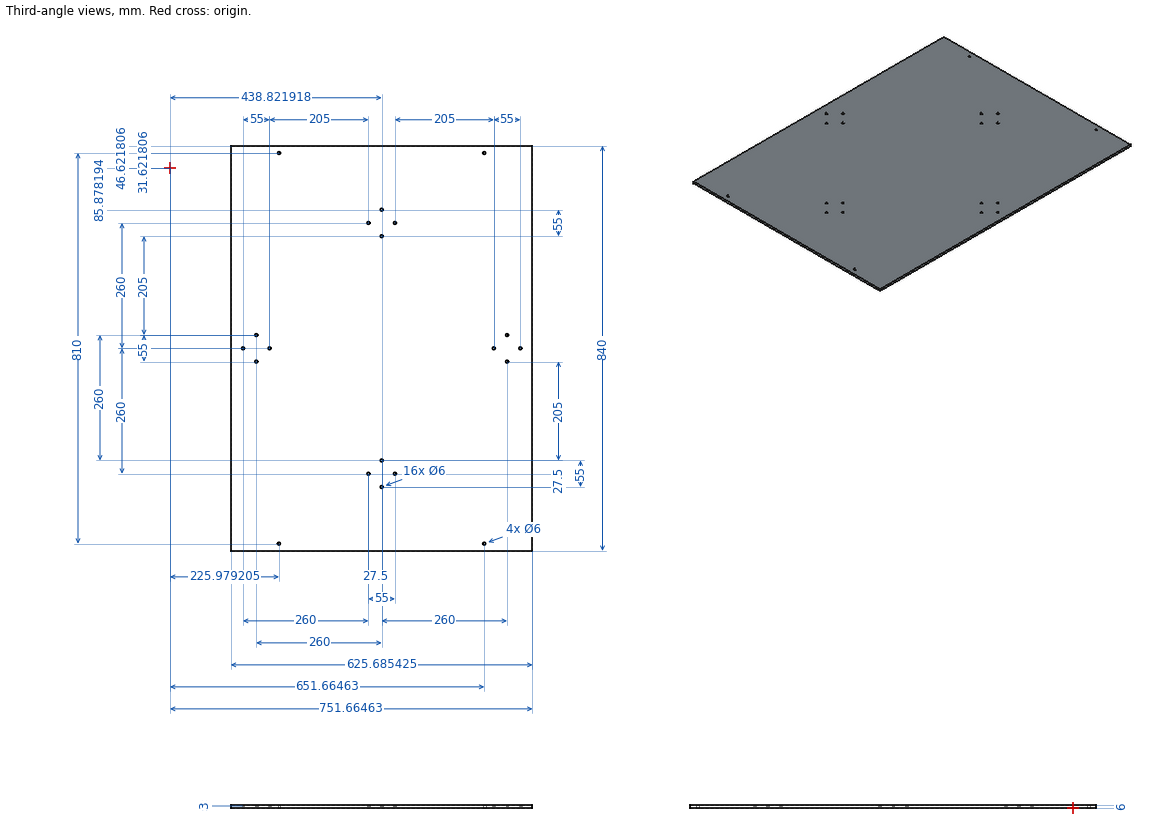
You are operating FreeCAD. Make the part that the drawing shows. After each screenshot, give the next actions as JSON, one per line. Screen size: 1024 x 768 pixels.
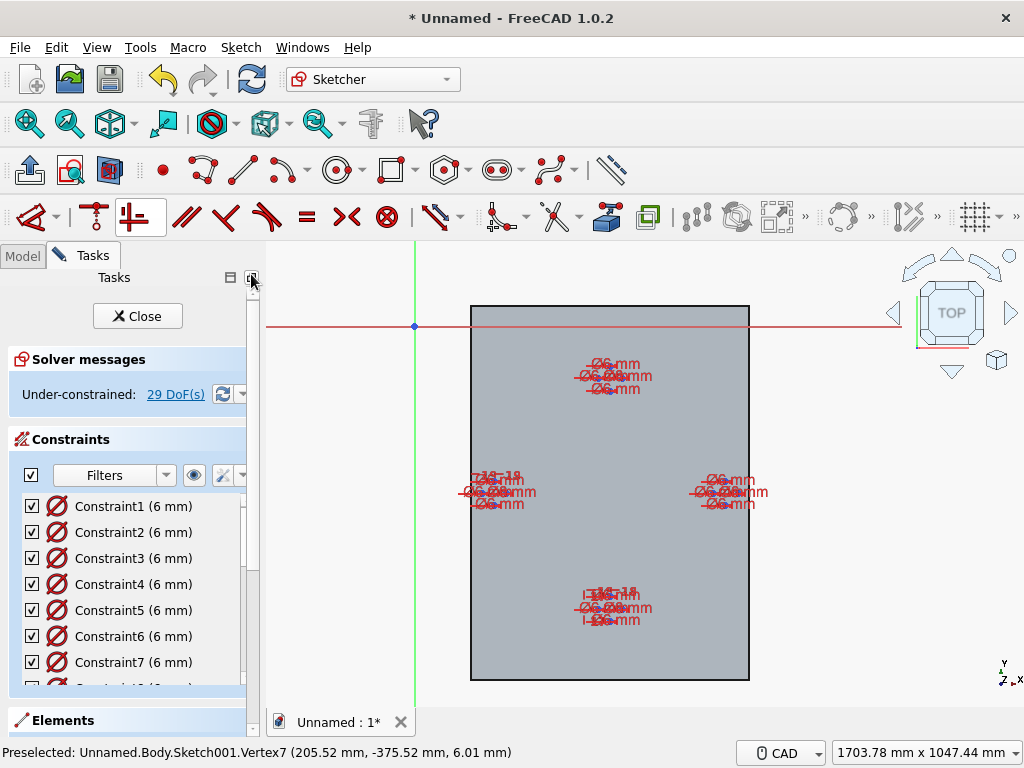
{"action": "left_click", "coordinate": [494, 482]}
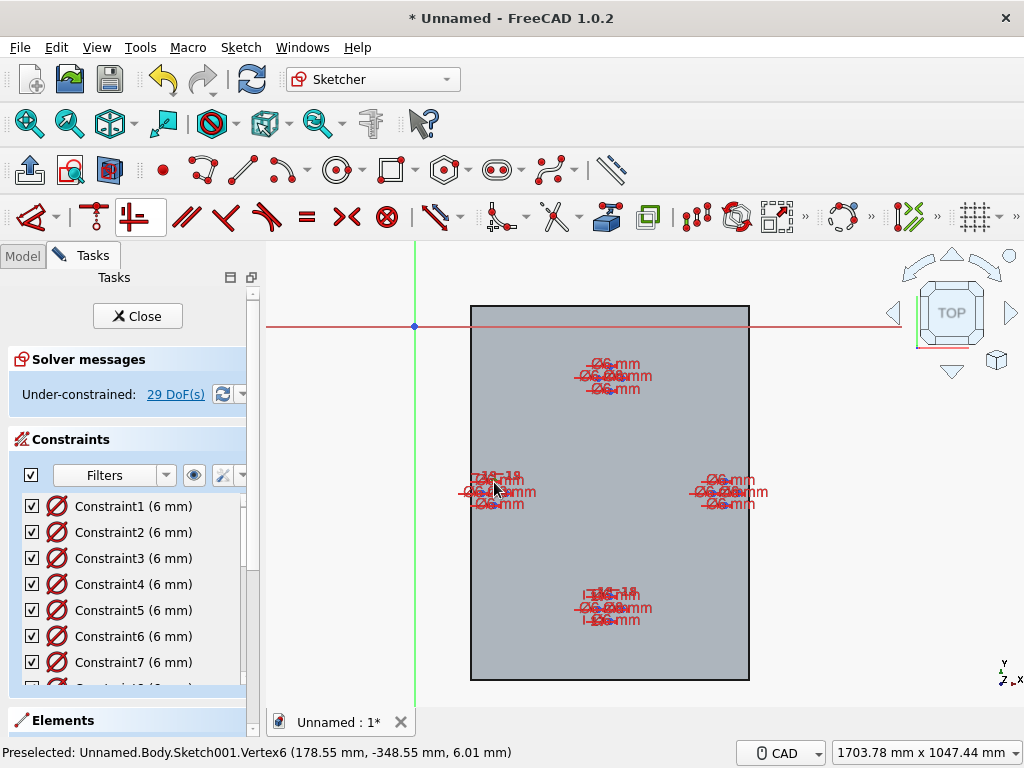
{"action": "left_click", "coordinate": [494, 506]}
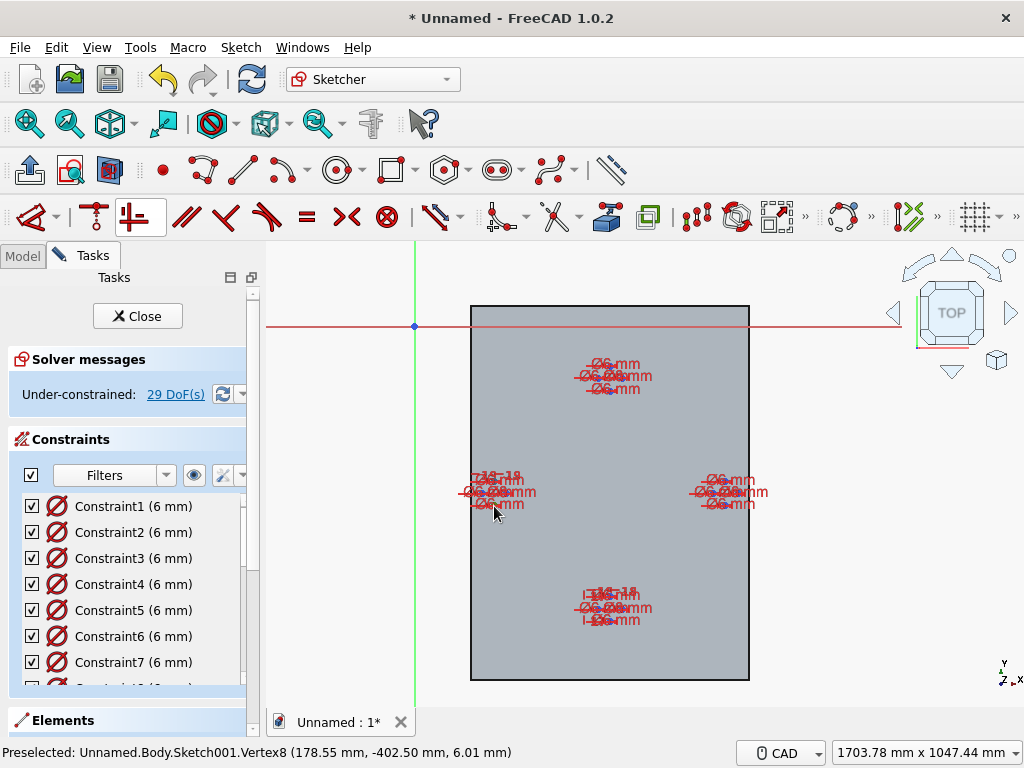
{"action": "key", "text": "v"}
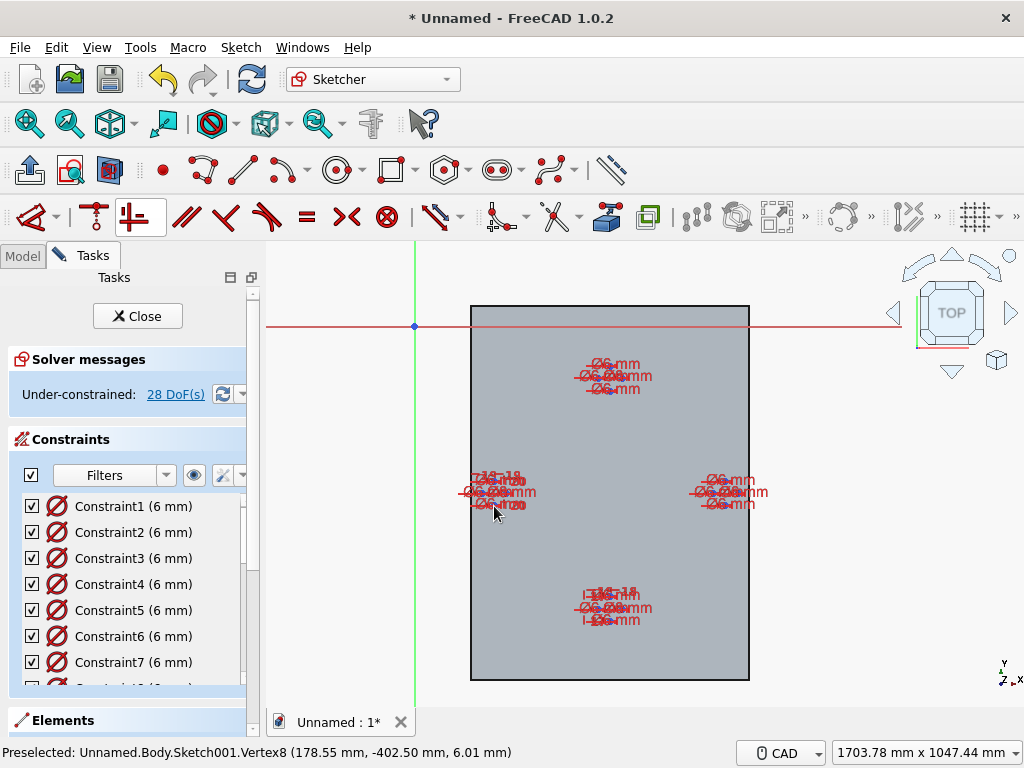
{"action": "left_click", "coordinate": [608, 599]}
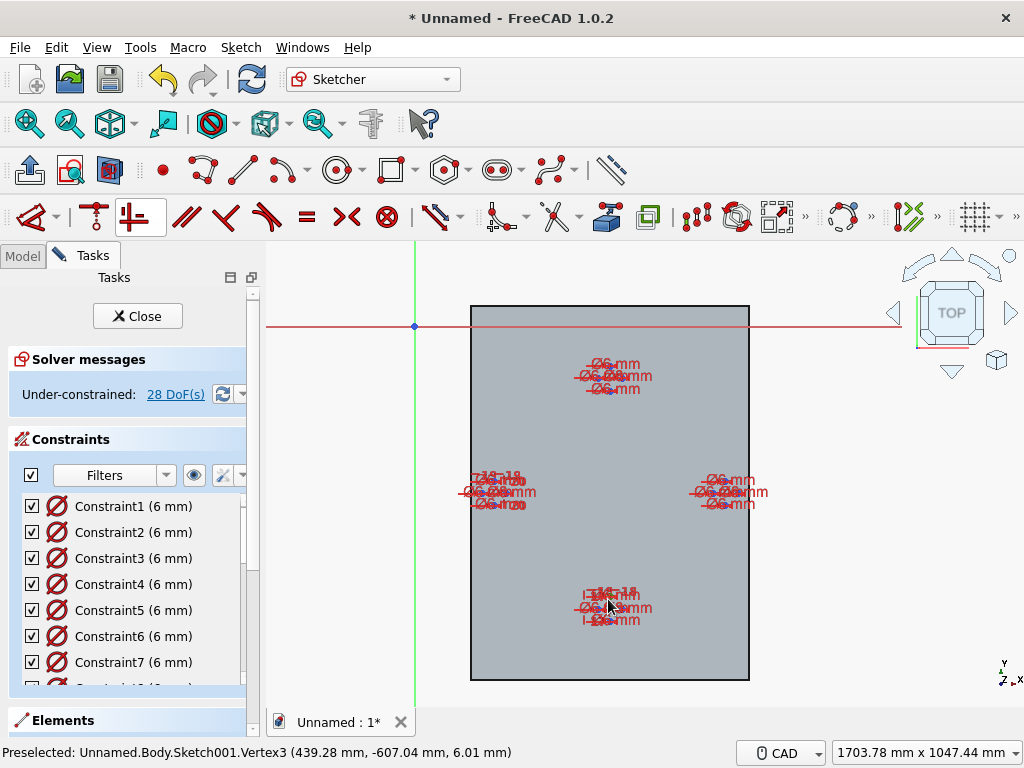
{"action": "left_click", "coordinate": [610, 391]}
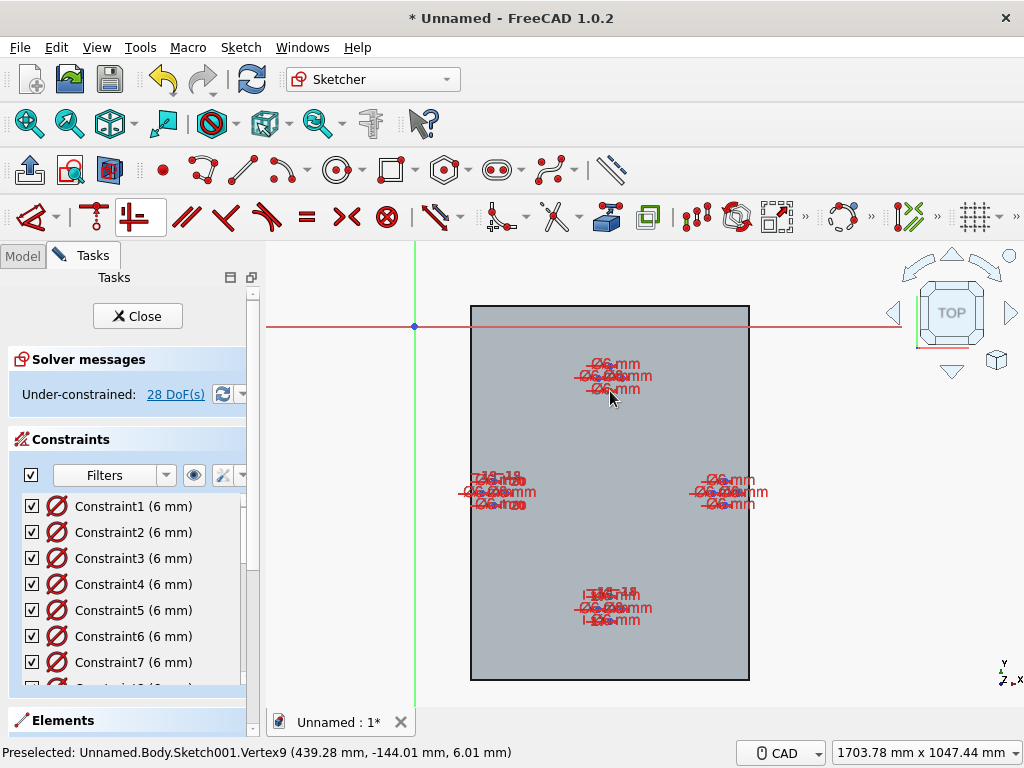
{"action": "left_click", "coordinate": [160, 218]}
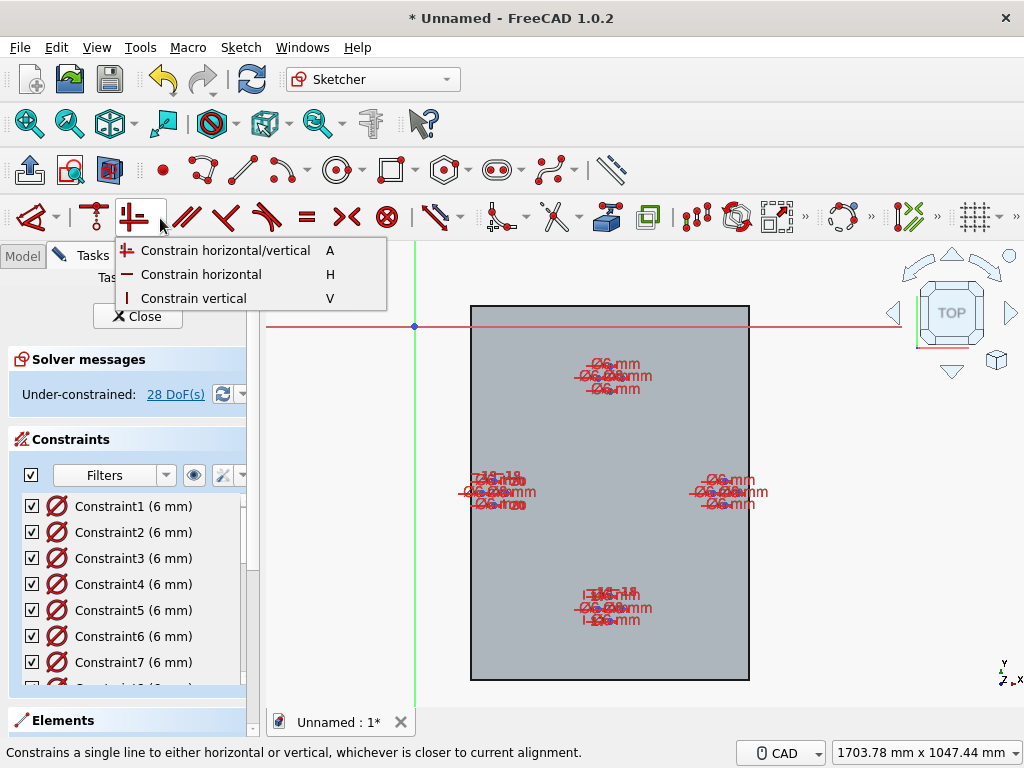
{"action": "left_click", "coordinate": [251, 298]}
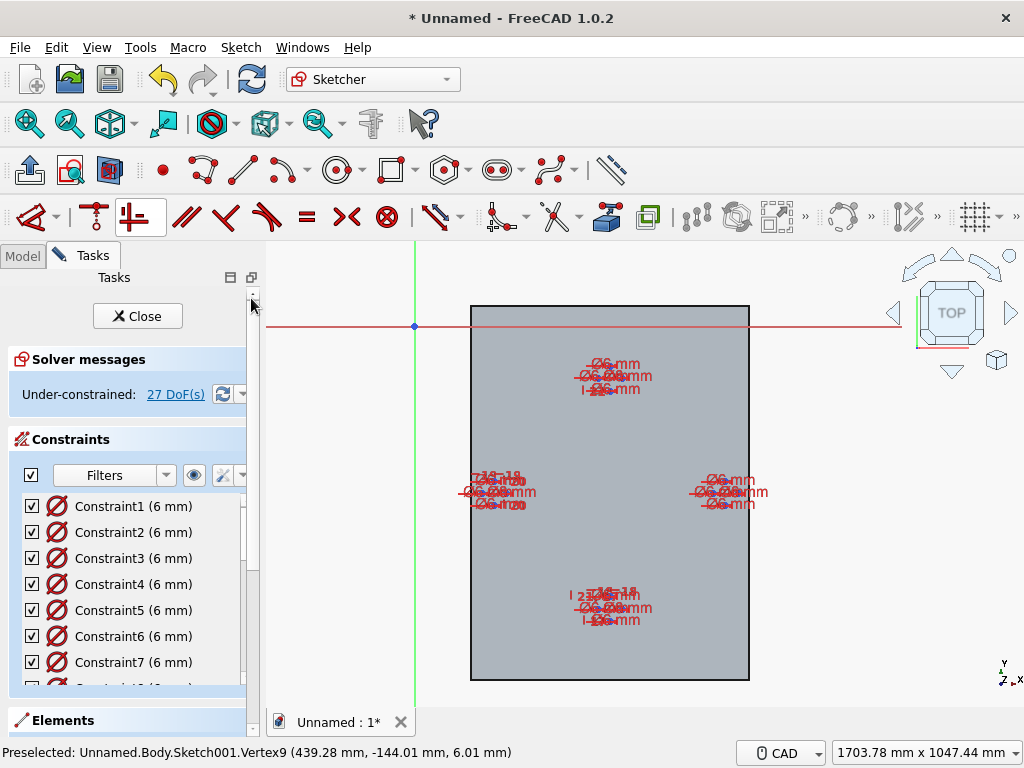
{"action": "left_click", "coordinate": [610, 391]}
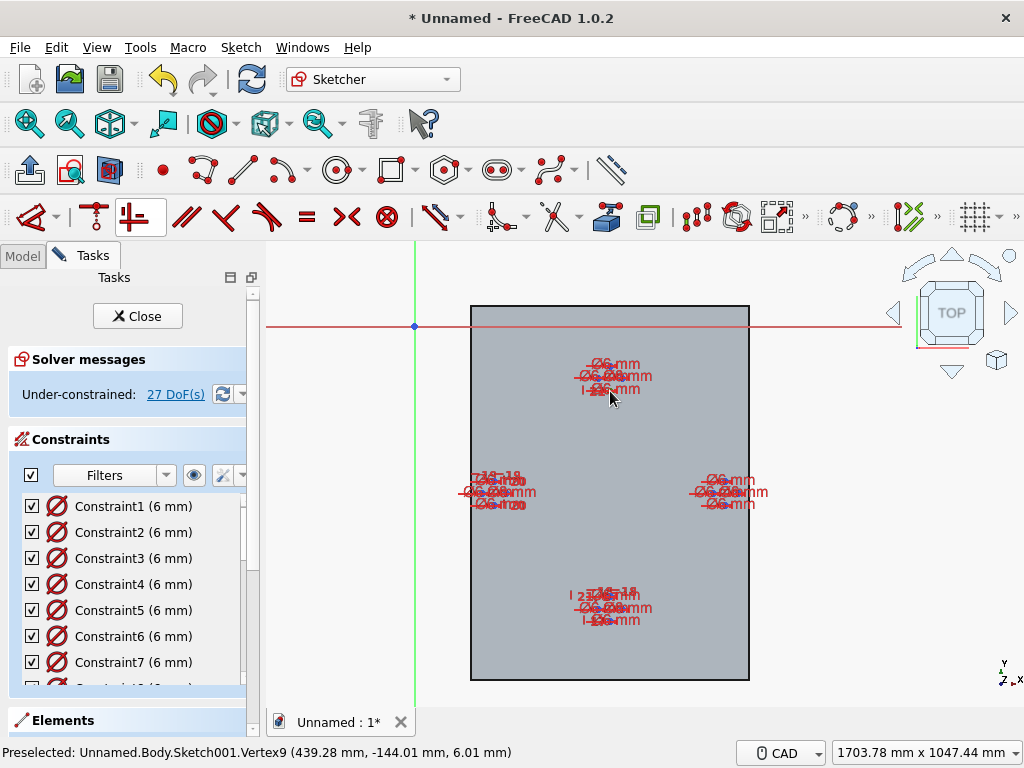
{"action": "left_click", "coordinate": [610, 366]}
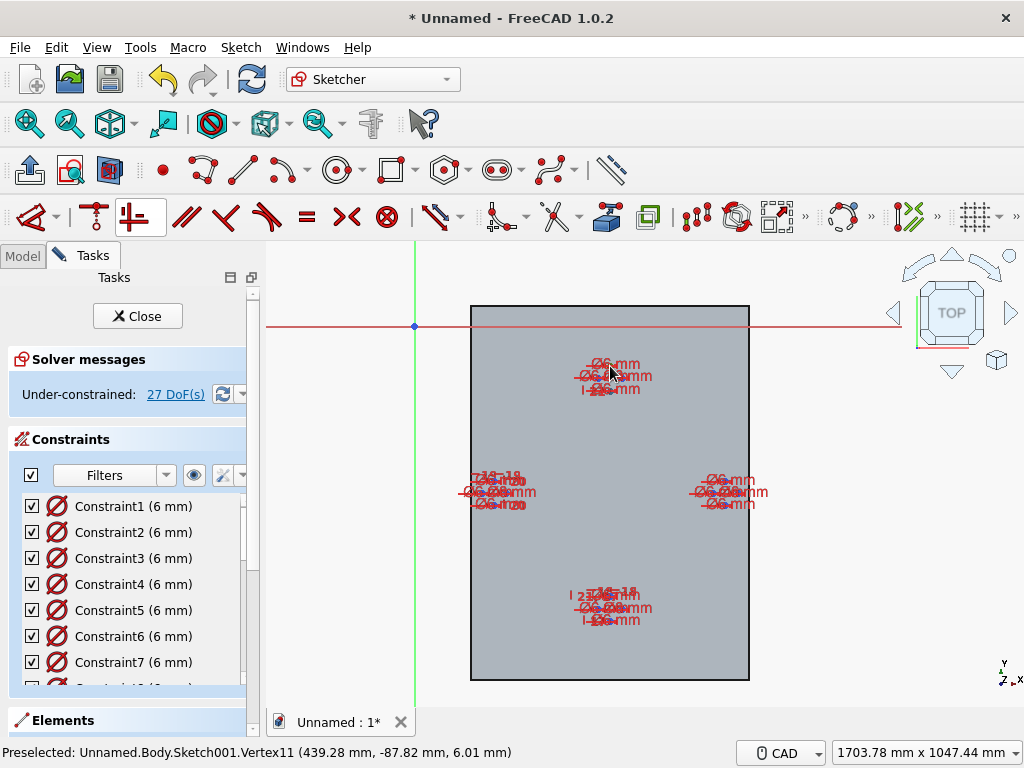
{"action": "left_click", "coordinate": [160, 218]}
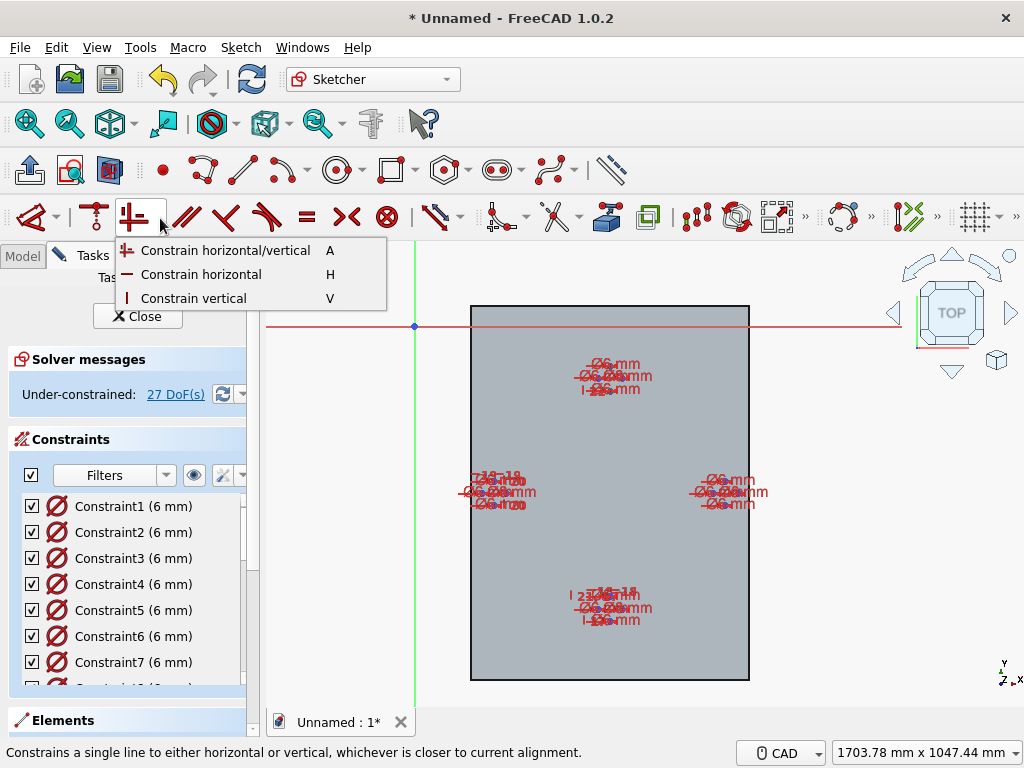
{"action": "left_click", "coordinate": [251, 298]}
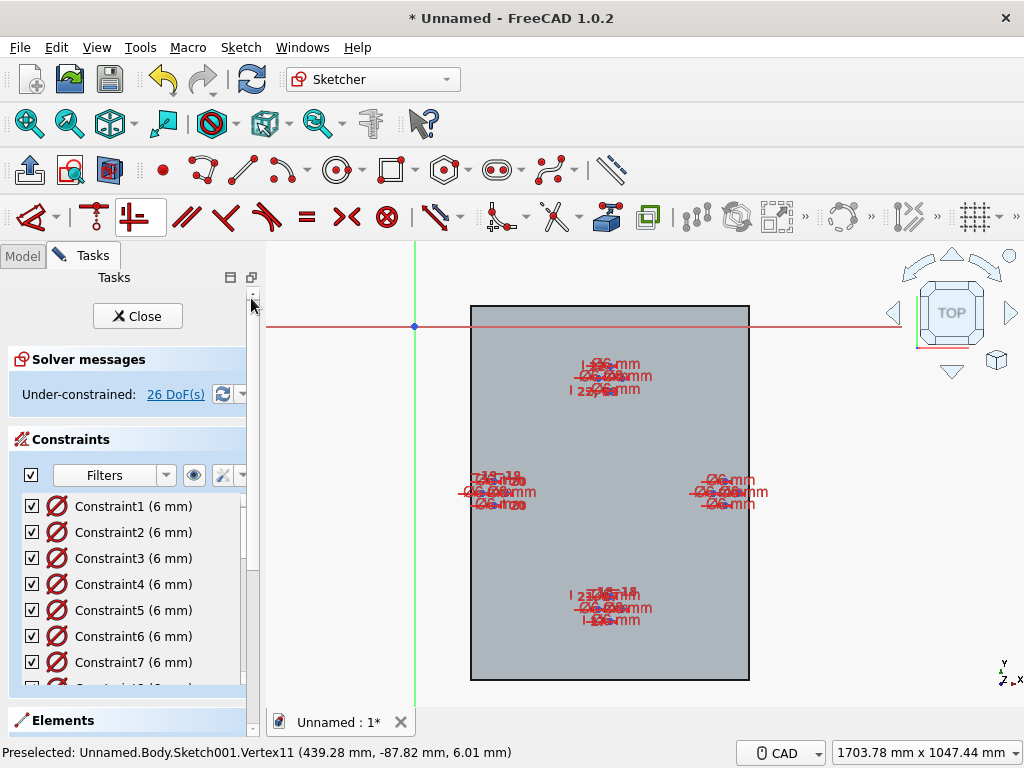
{"action": "left_click", "coordinate": [598, 378]}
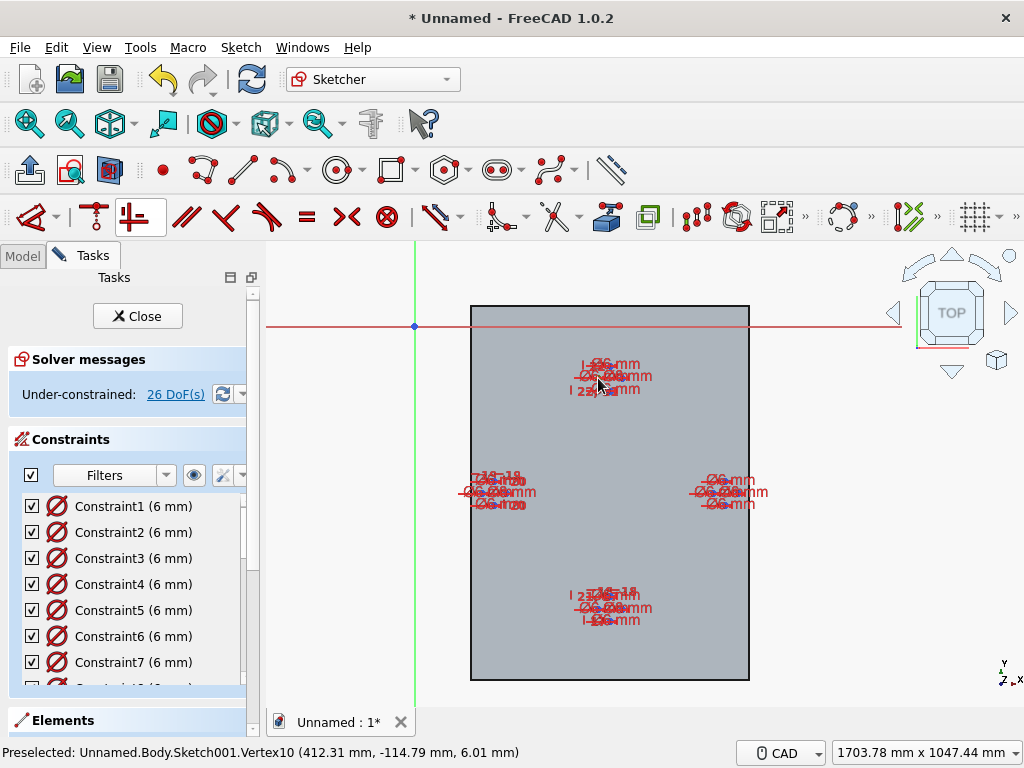
{"action": "left_click", "coordinate": [622, 378]}